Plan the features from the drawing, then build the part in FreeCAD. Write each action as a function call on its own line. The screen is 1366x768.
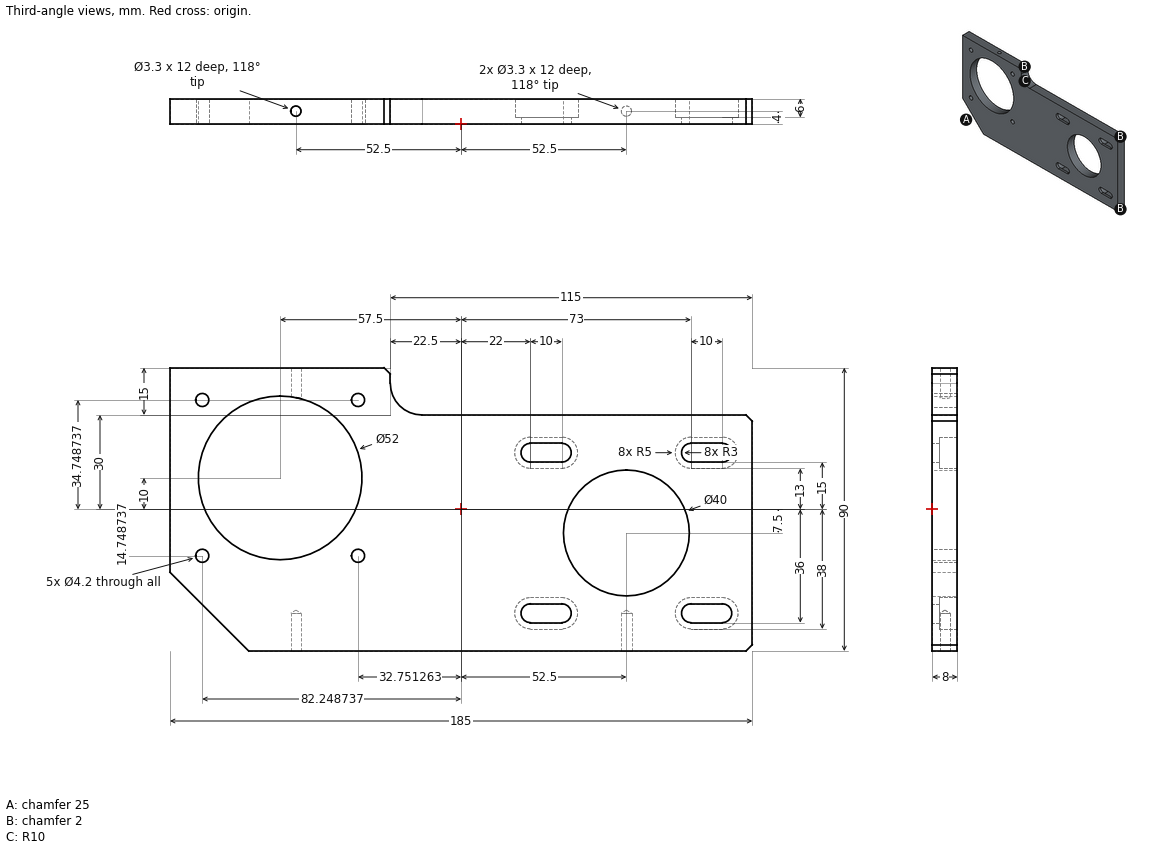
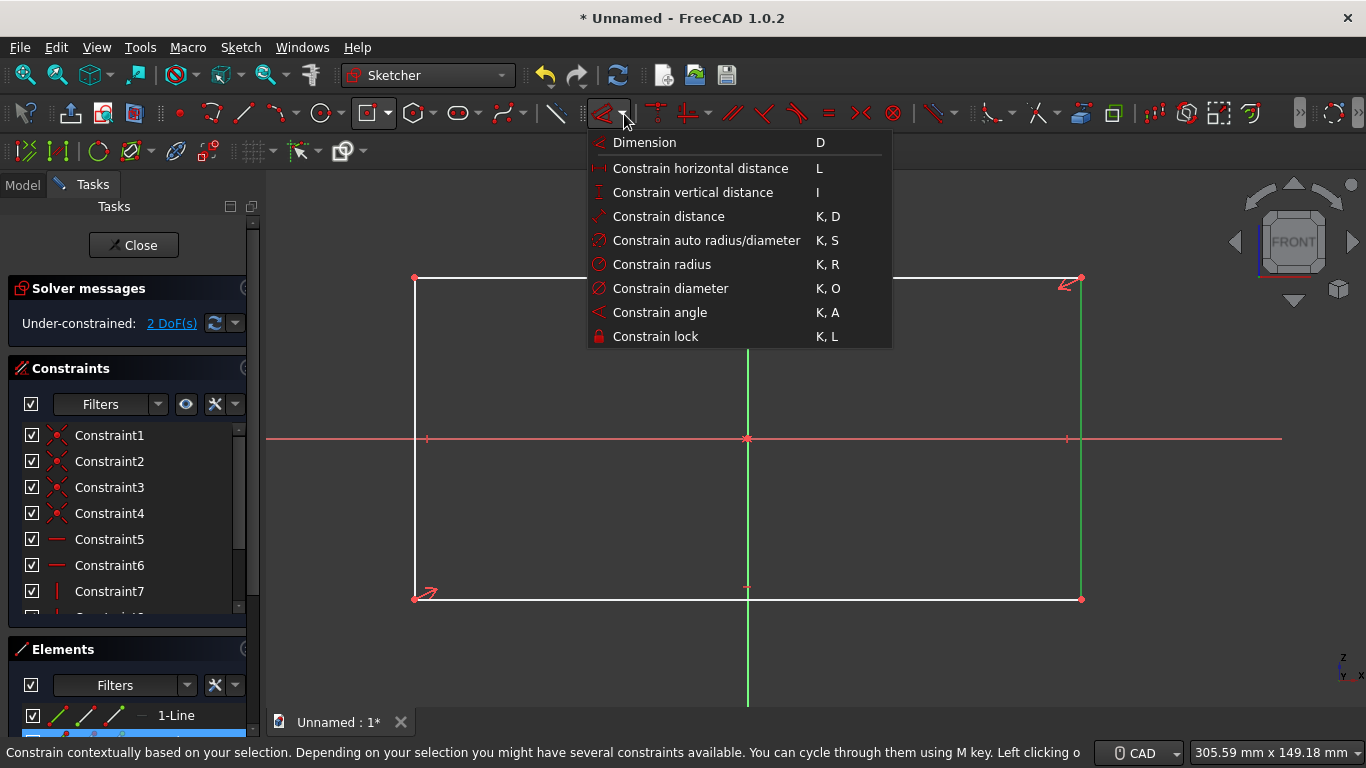
click(740, 192)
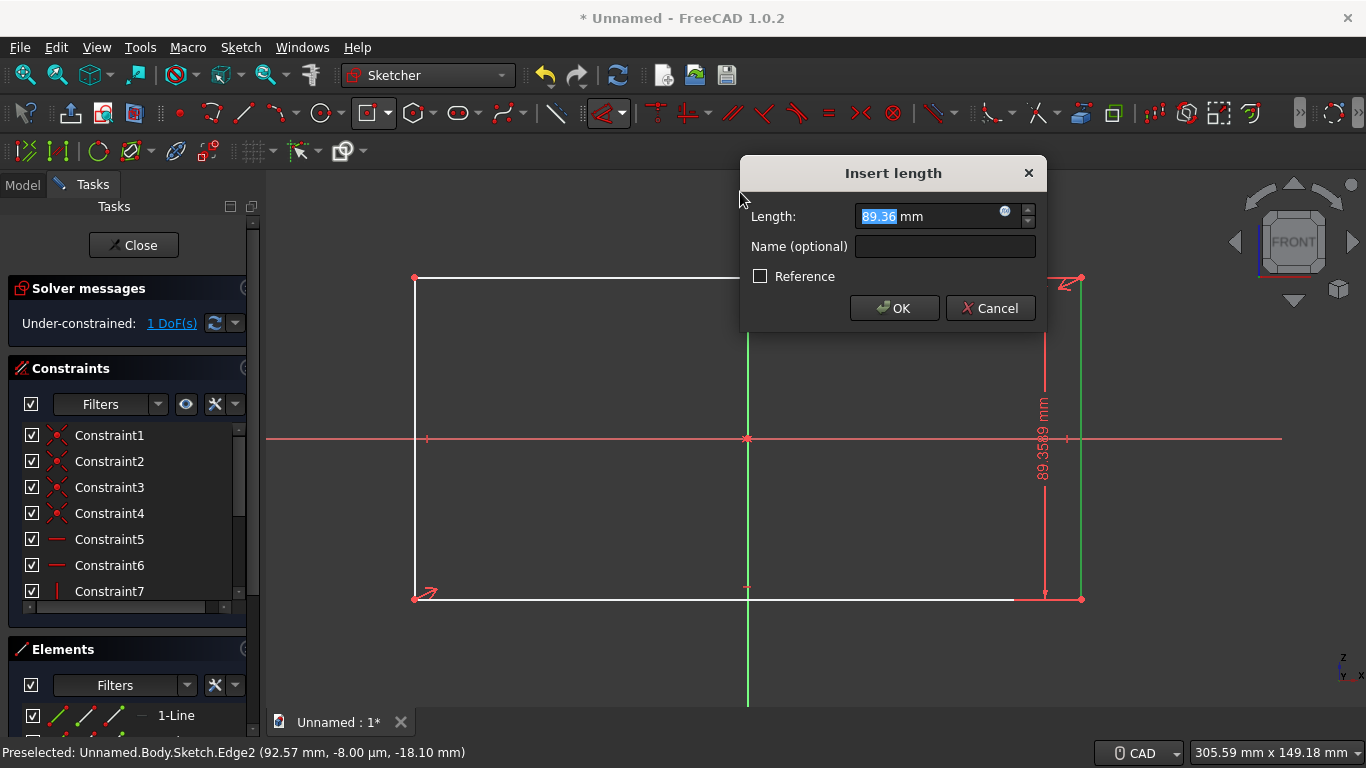
text(90)
key(Return)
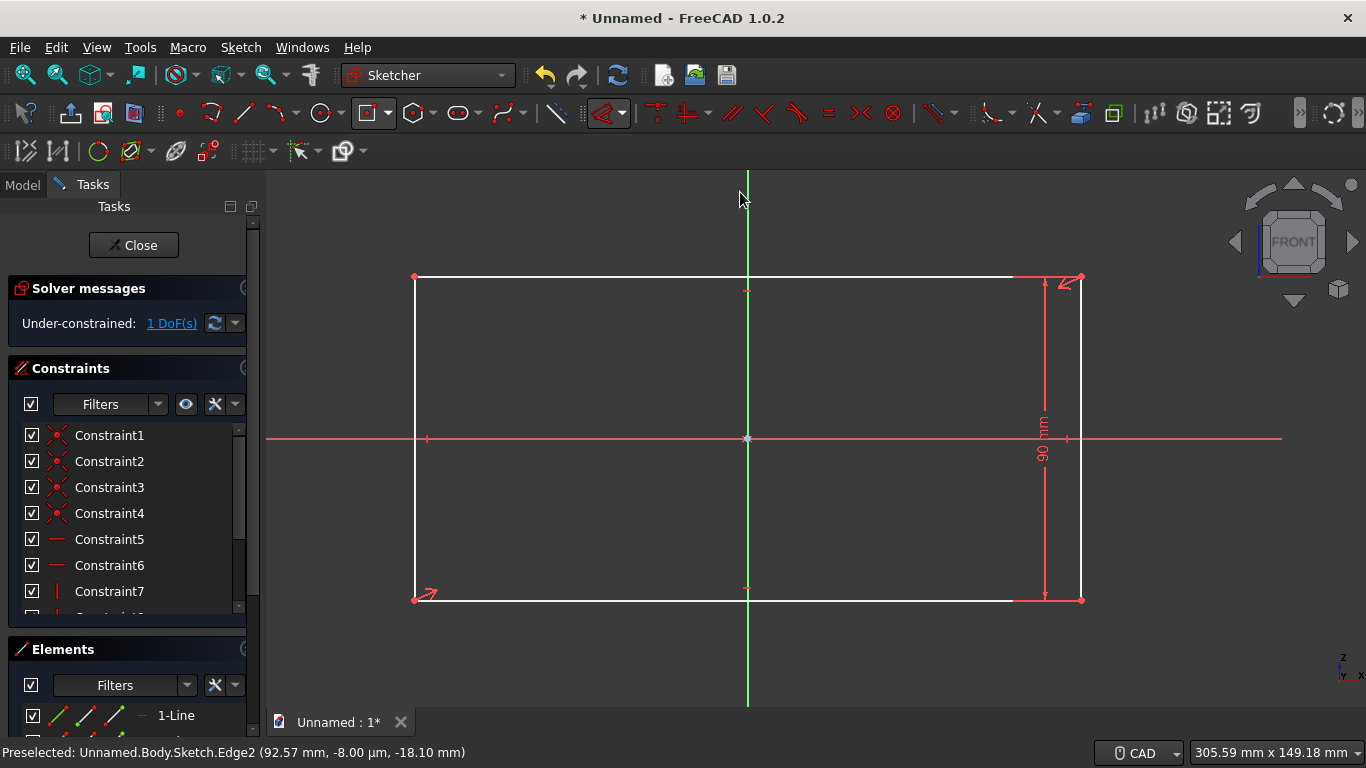
click(614, 601)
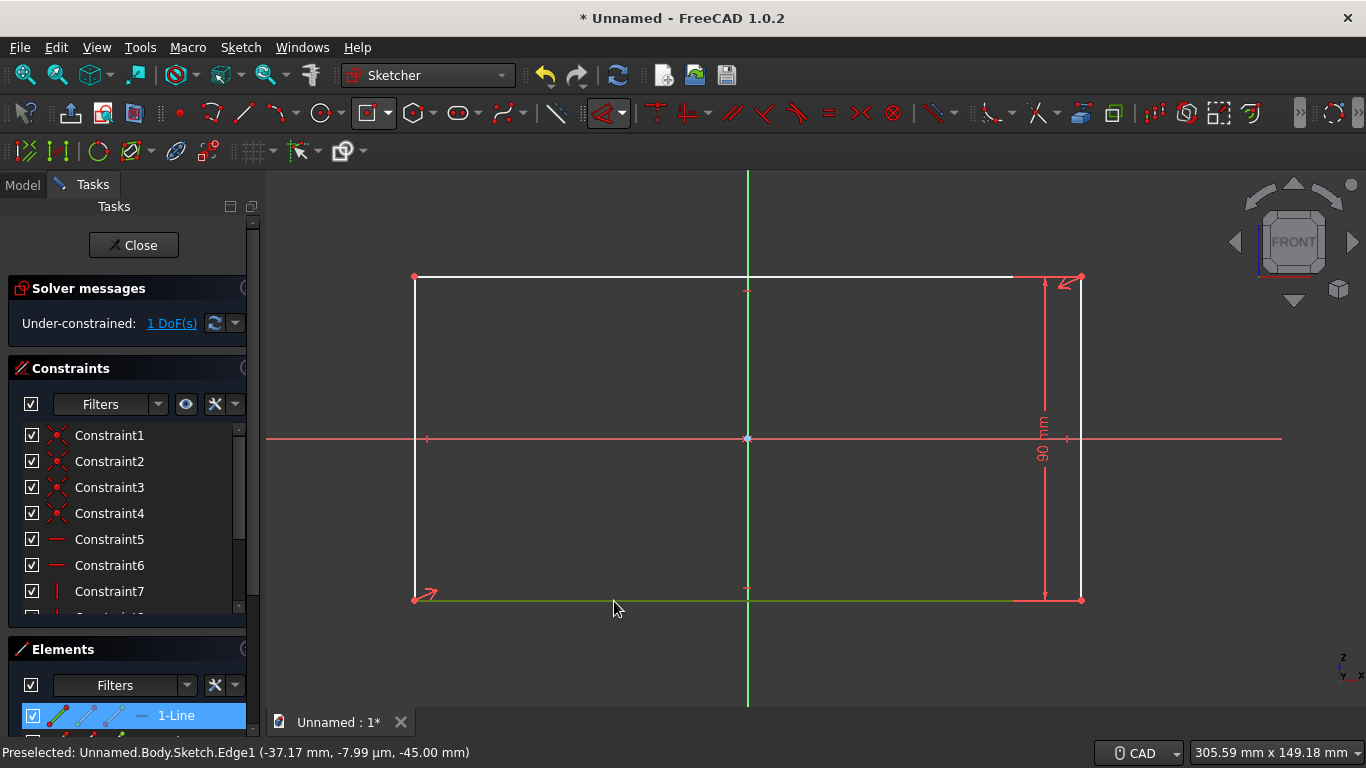
click(624, 114)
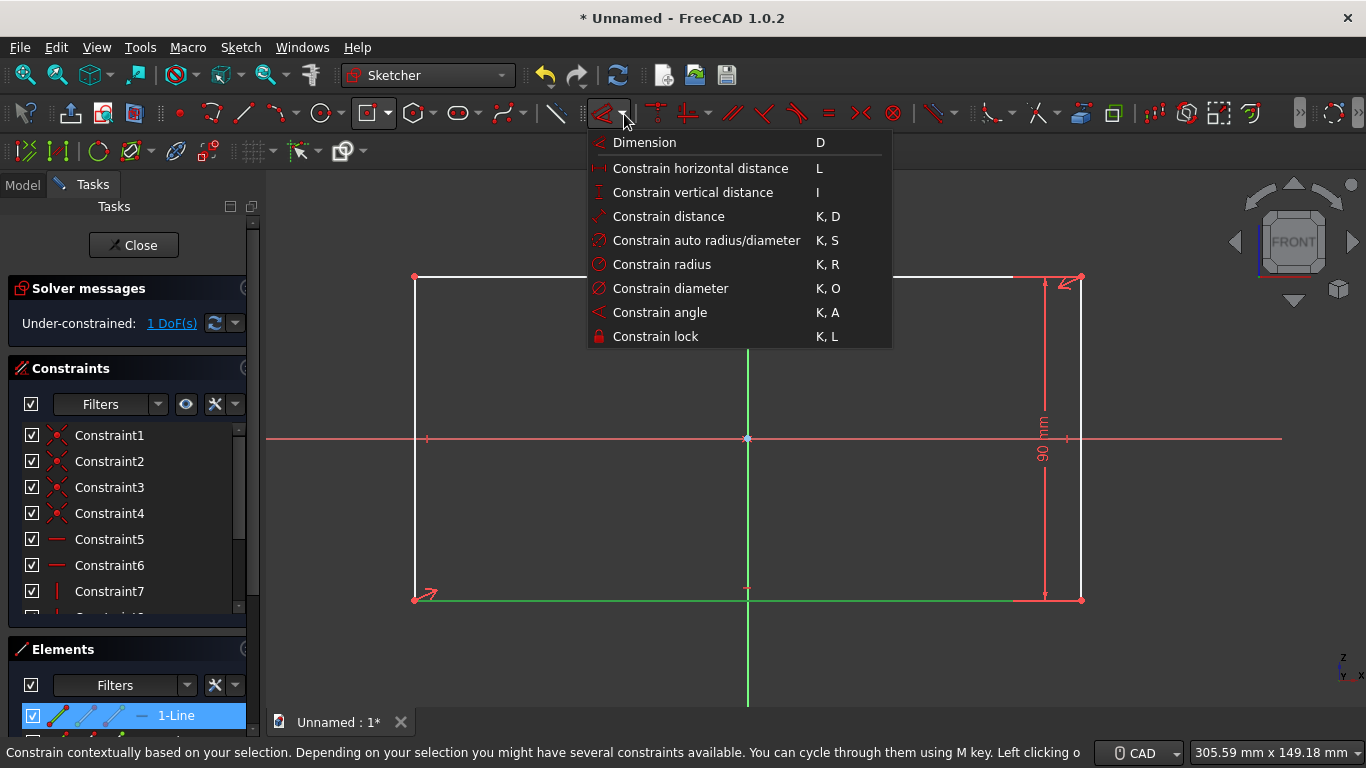
click(740, 168)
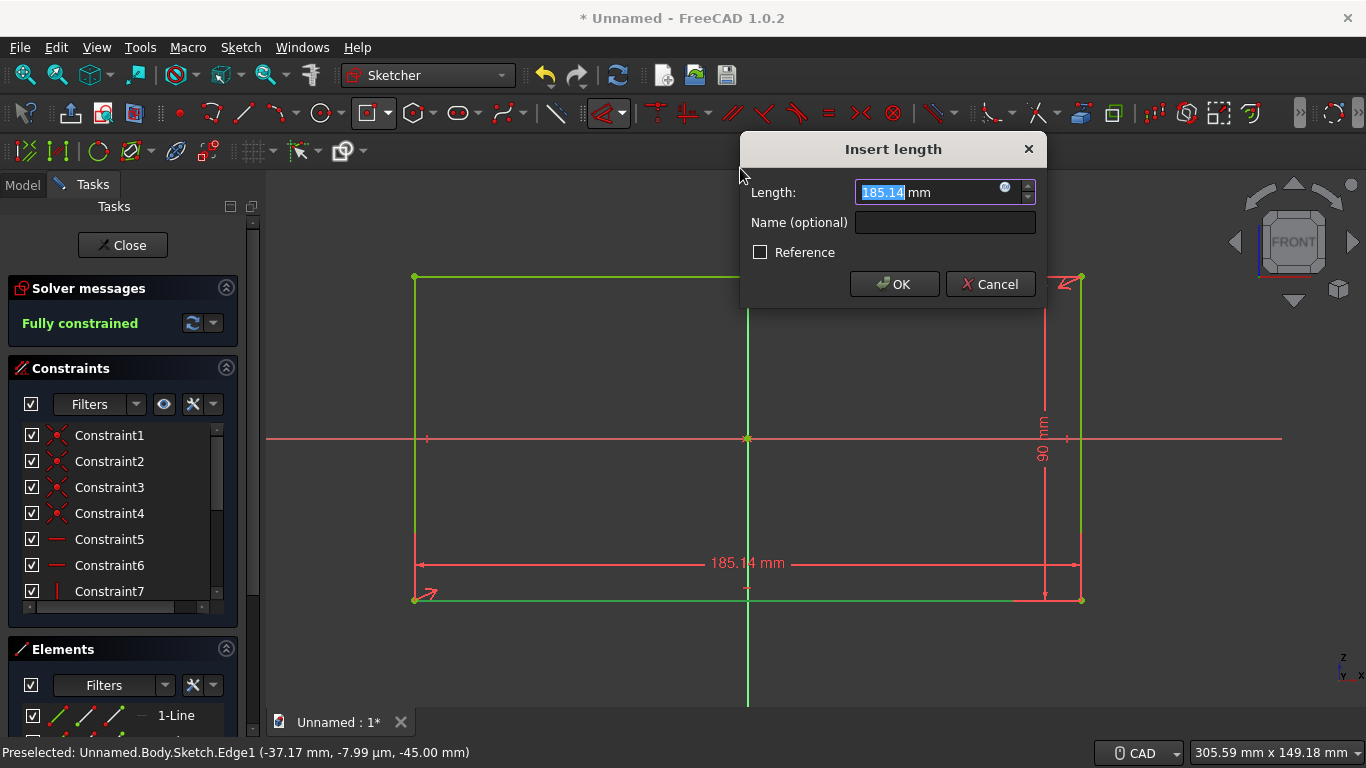
text(185)
key(Return)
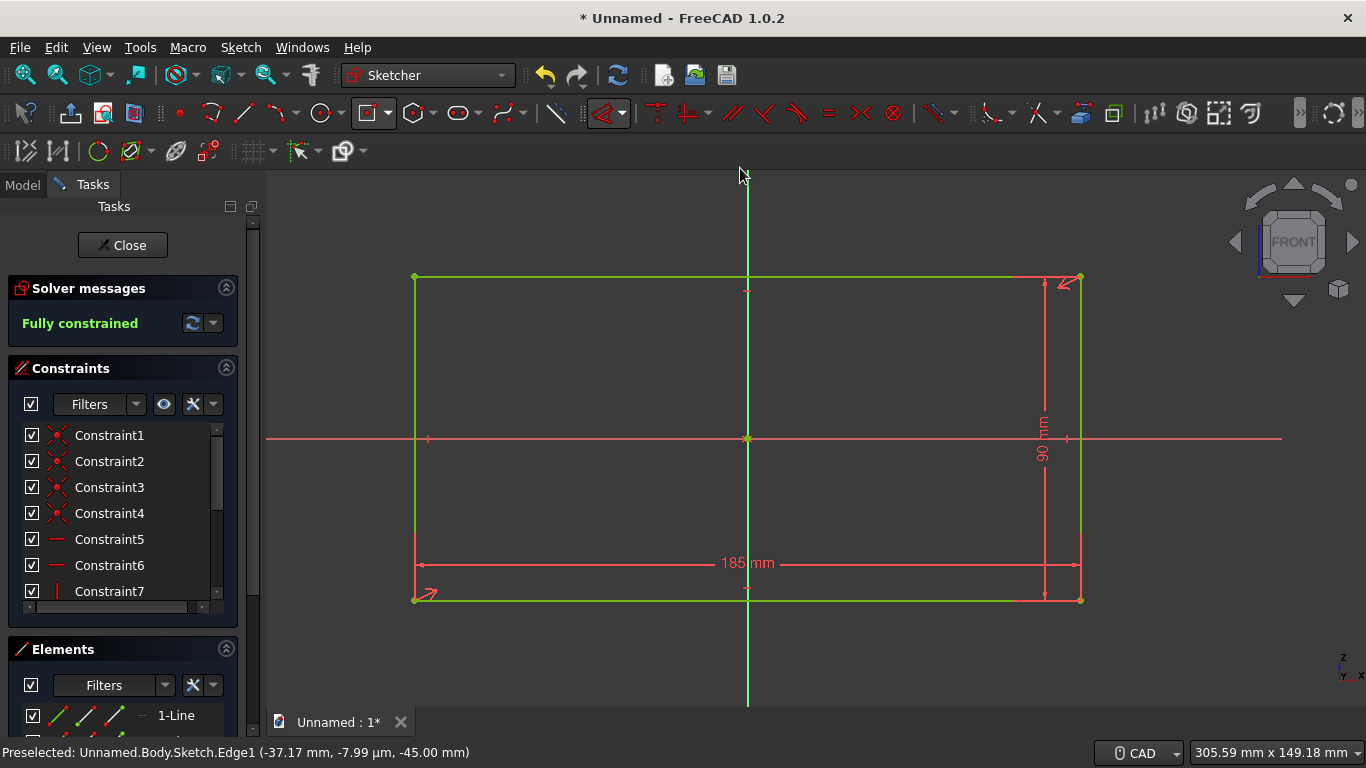
click(123, 245)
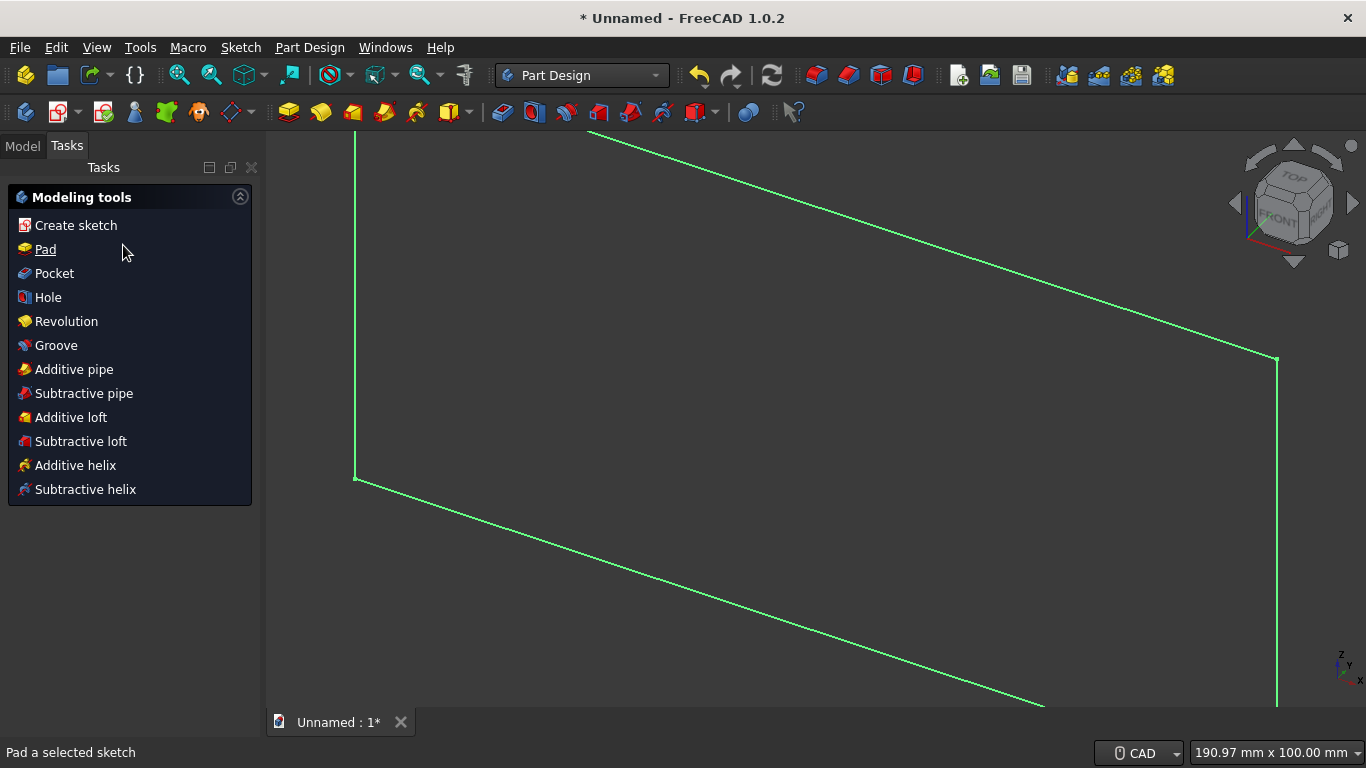
click(290, 112)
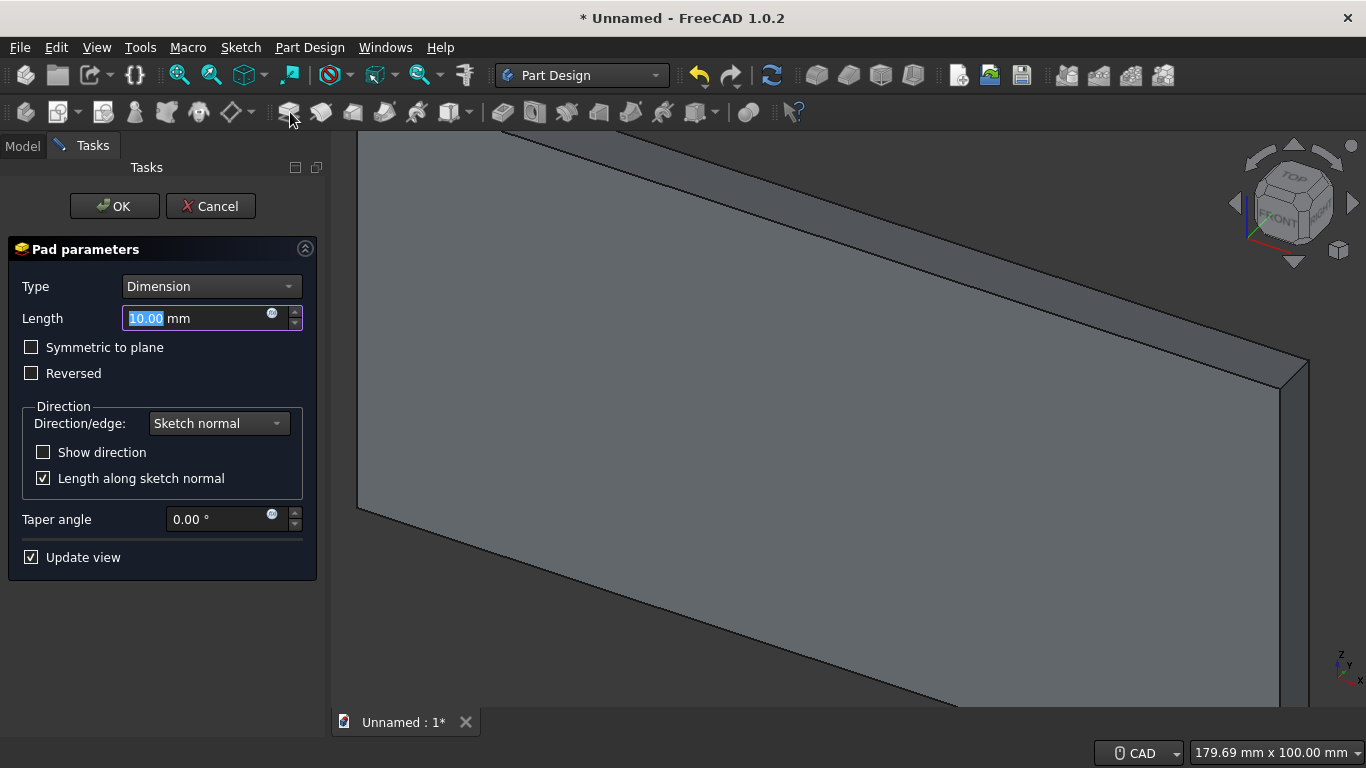
text(8)
key(Tab)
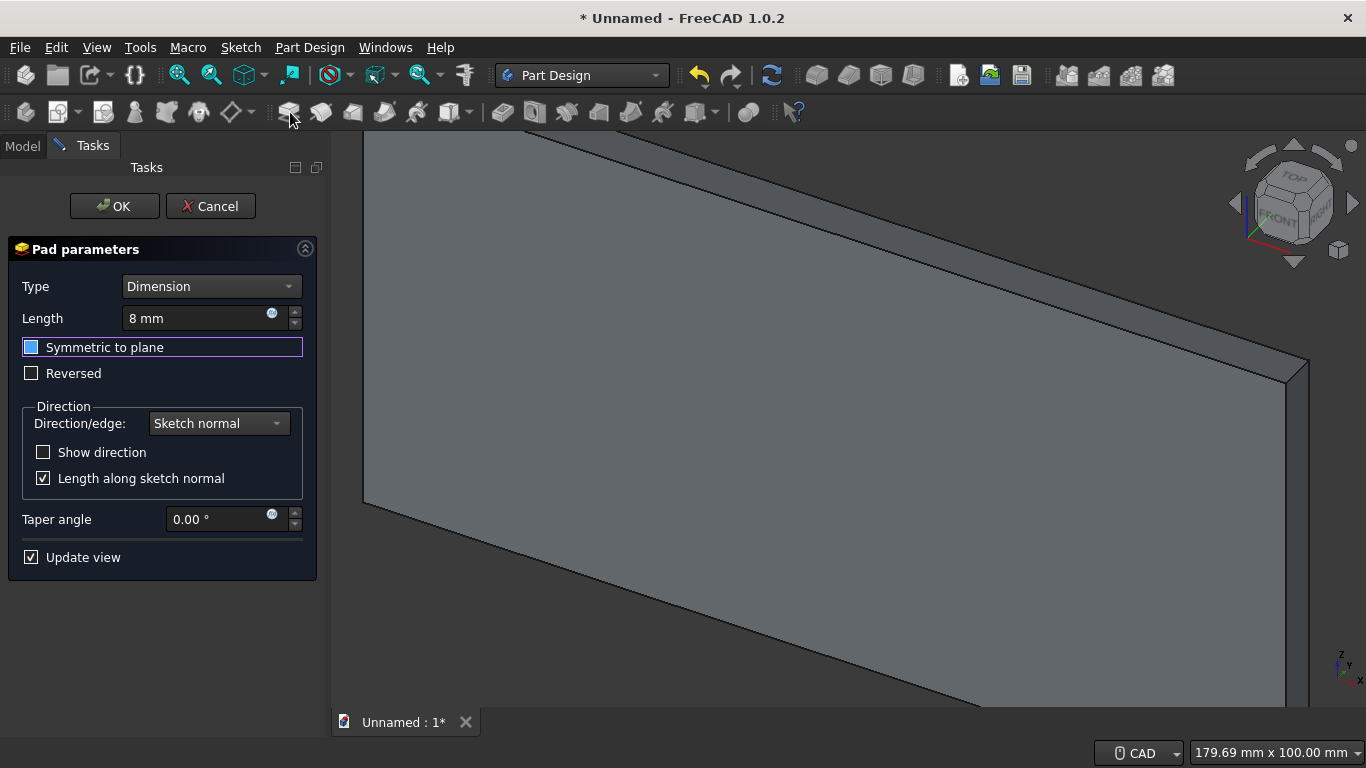
click(30, 373)